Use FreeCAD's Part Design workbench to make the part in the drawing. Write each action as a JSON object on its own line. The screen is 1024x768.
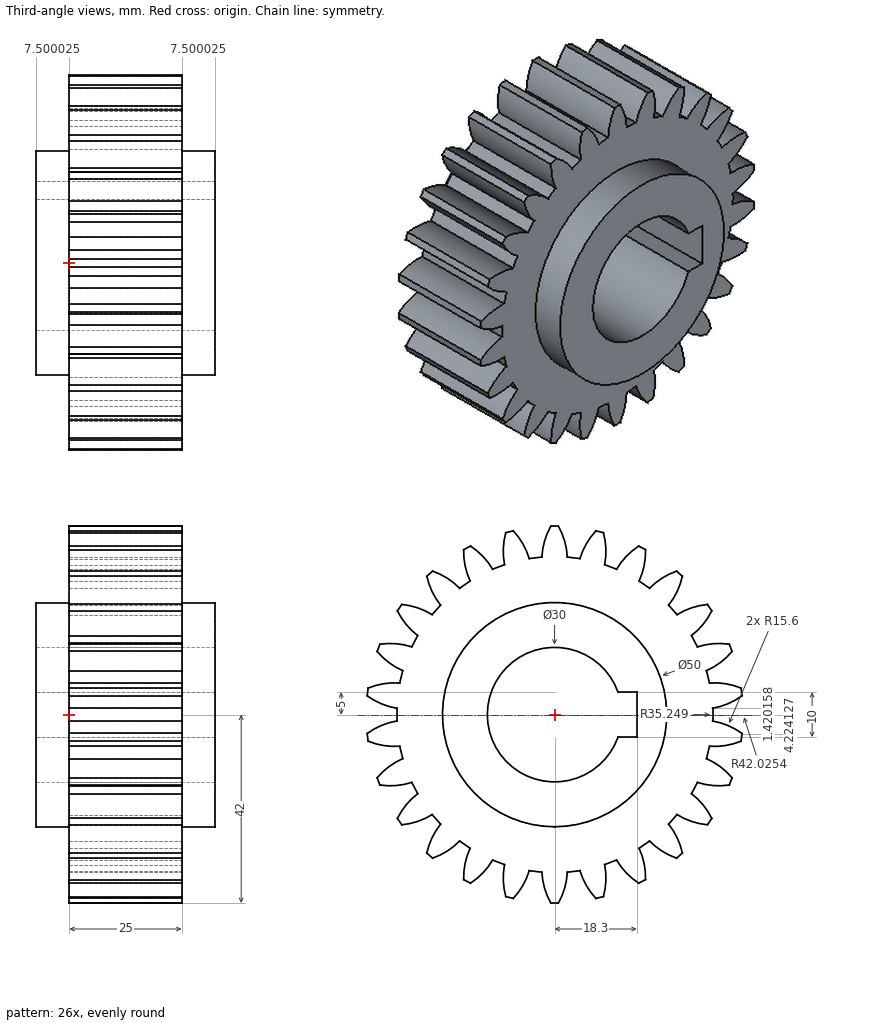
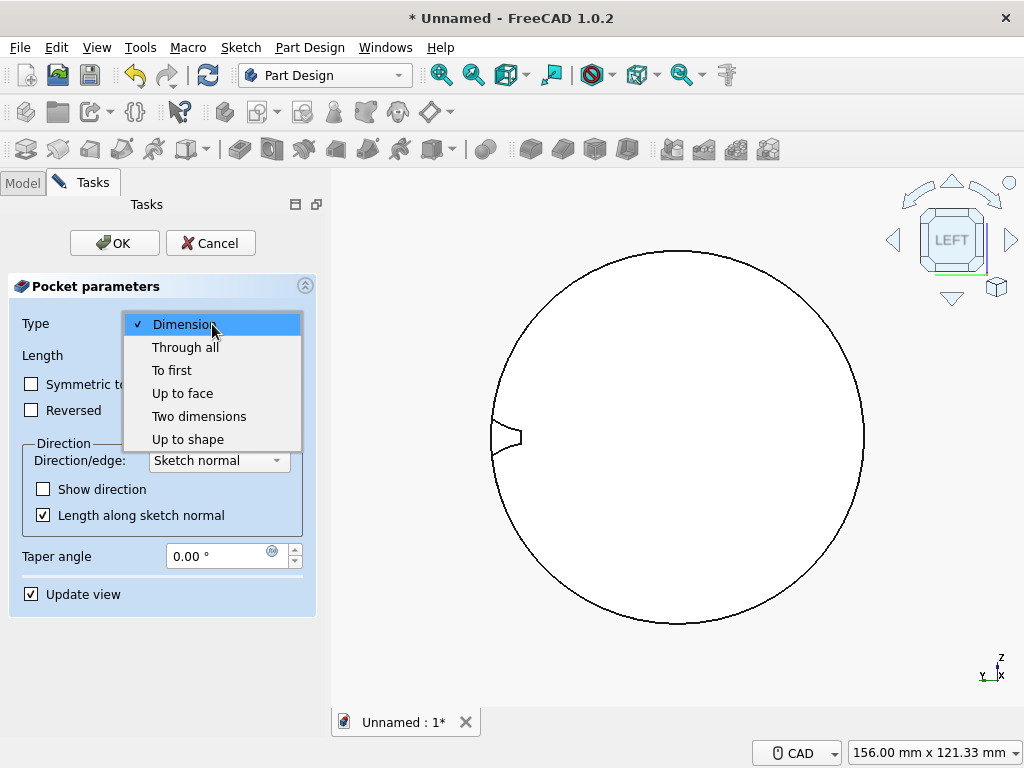
{"action": "left_click", "coordinate": [212, 348]}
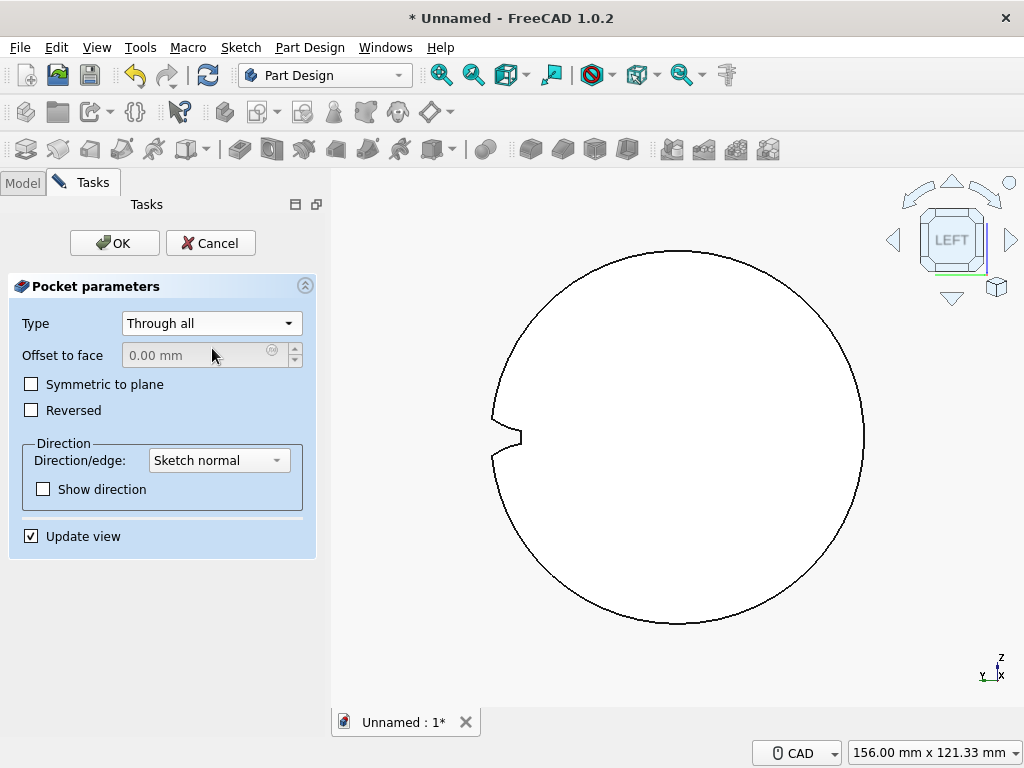
{"action": "left_click", "coordinate": [115, 243]}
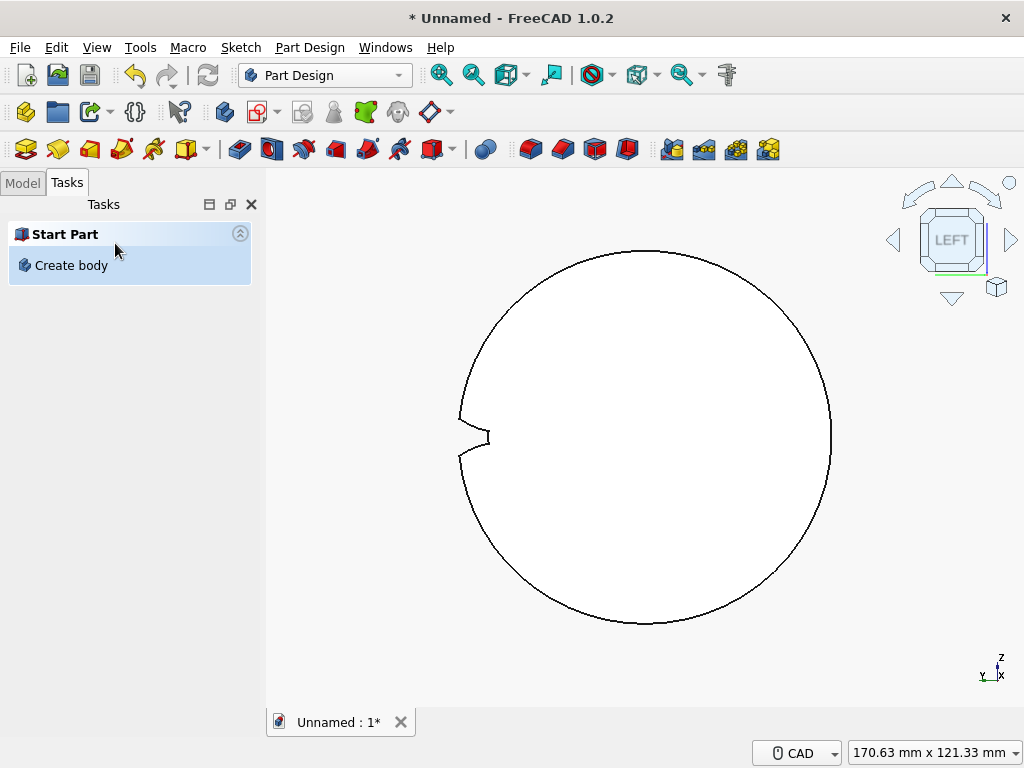
{"action": "left_click", "coordinate": [23, 182]}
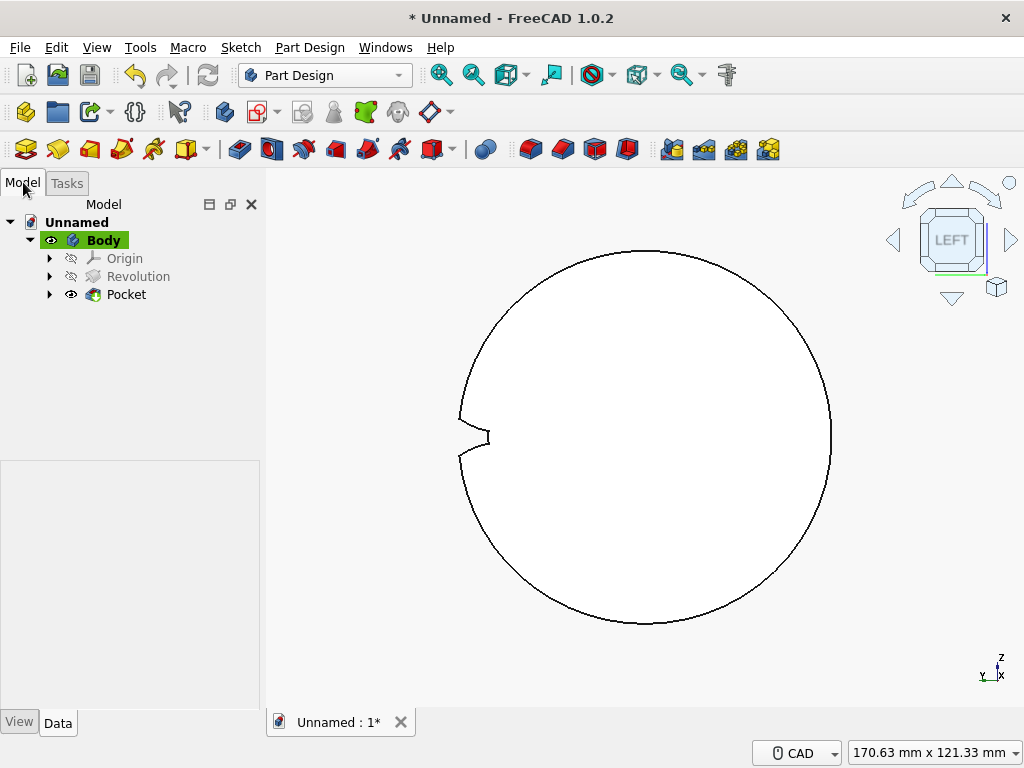
{"action": "left_click", "coordinate": [116, 294]}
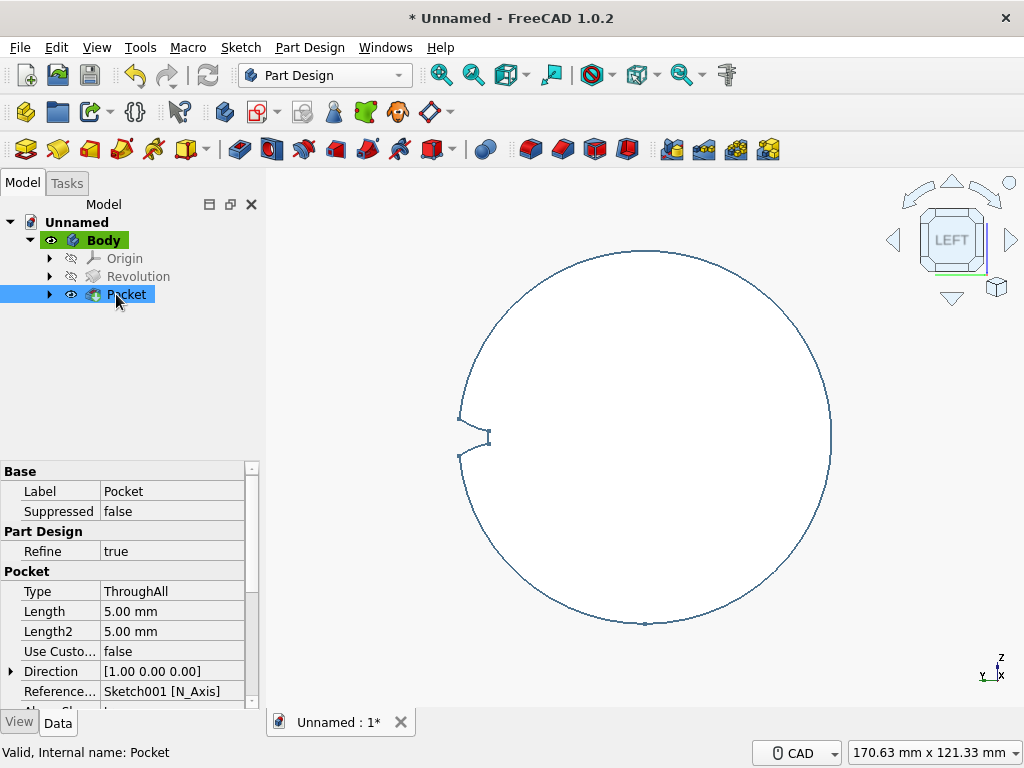
{"action": "left_click", "coordinate": [736, 150]}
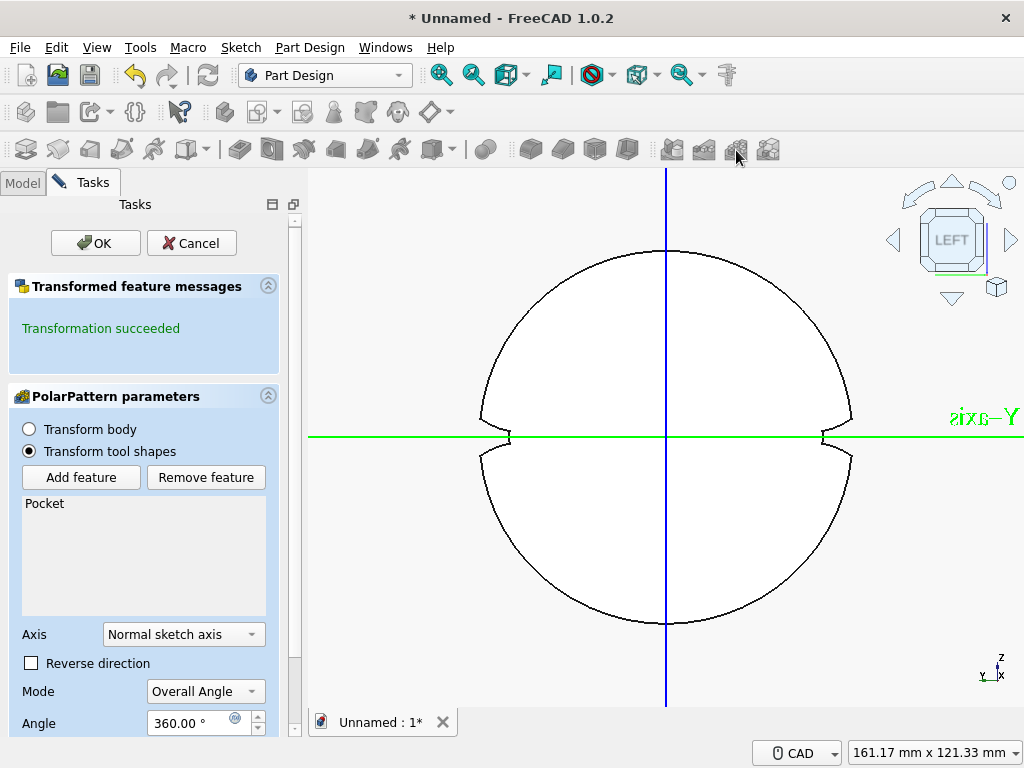
{"action": "left_click", "coordinate": [184, 634]}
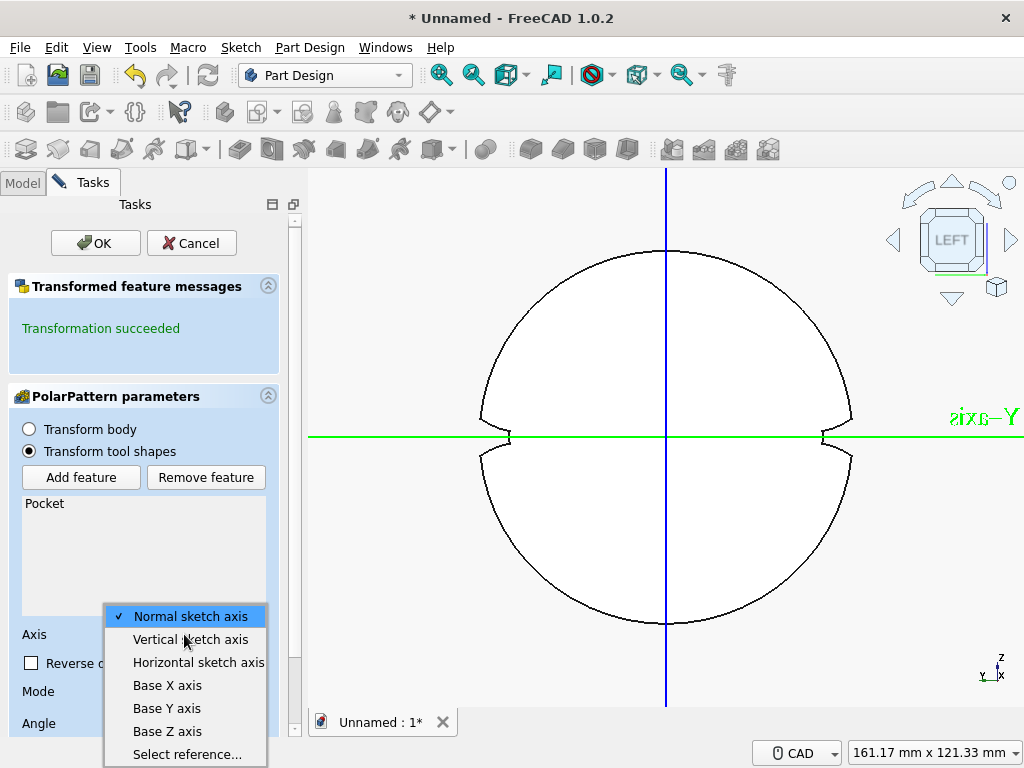
{"action": "left_click", "coordinate": [184, 686]}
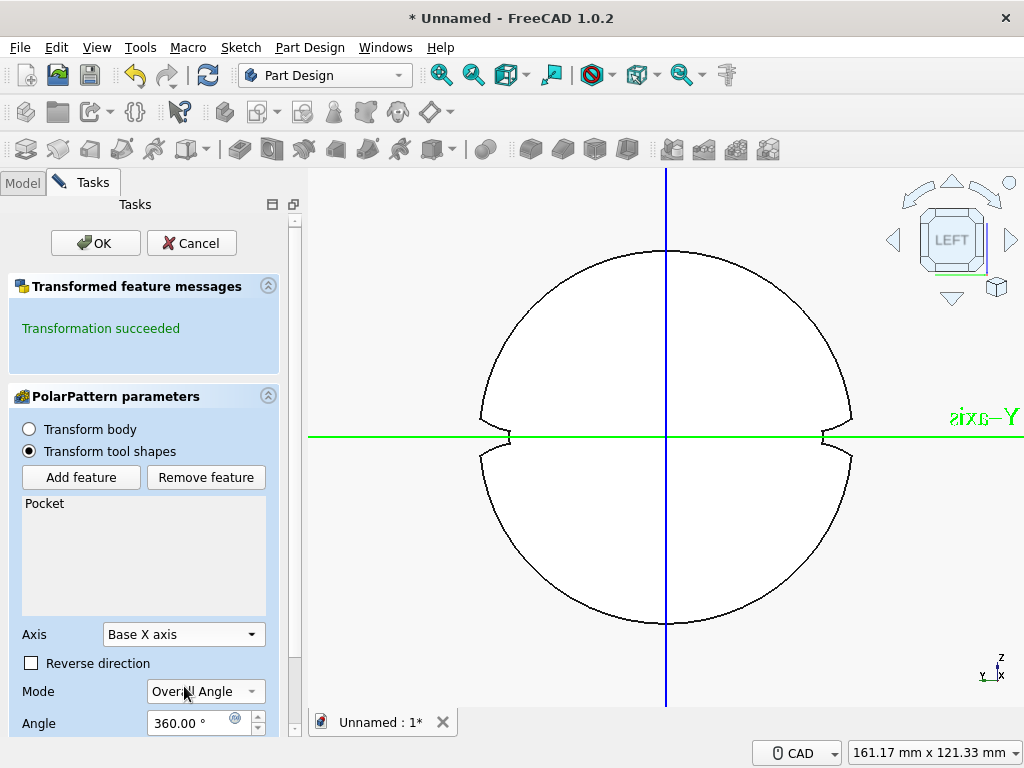
{"action": "scroll", "coordinate": [295, 475], "scroll_direction": "down", "scroll_amount": 2}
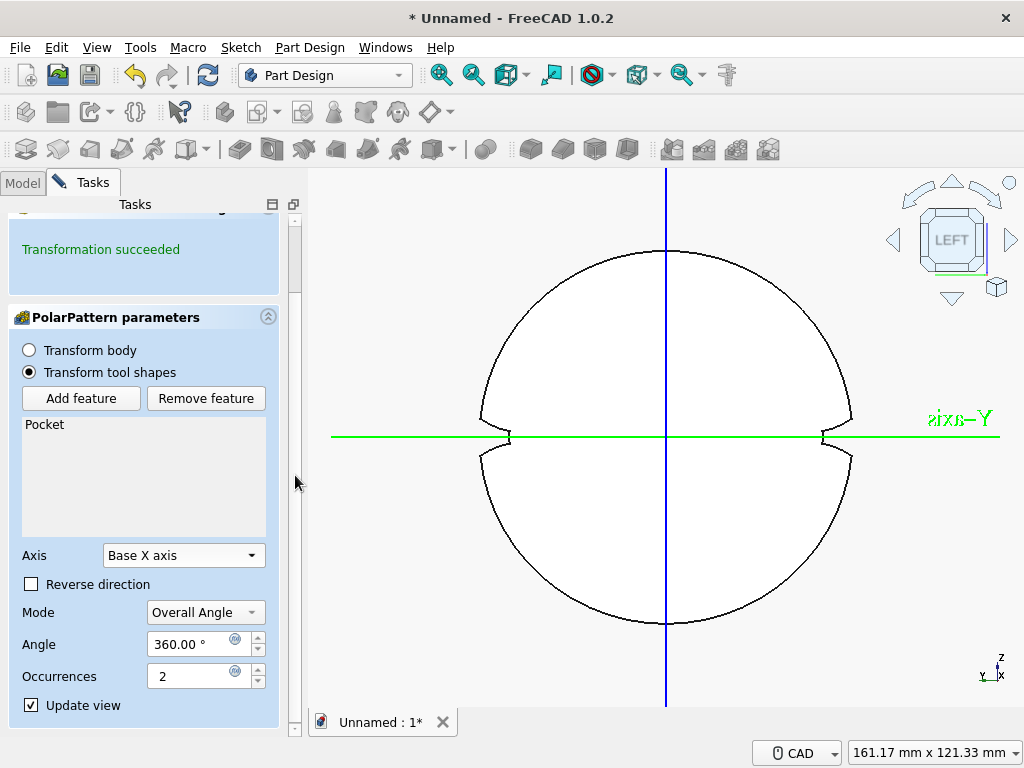
{"action": "triple_click", "coordinate": [198, 676]}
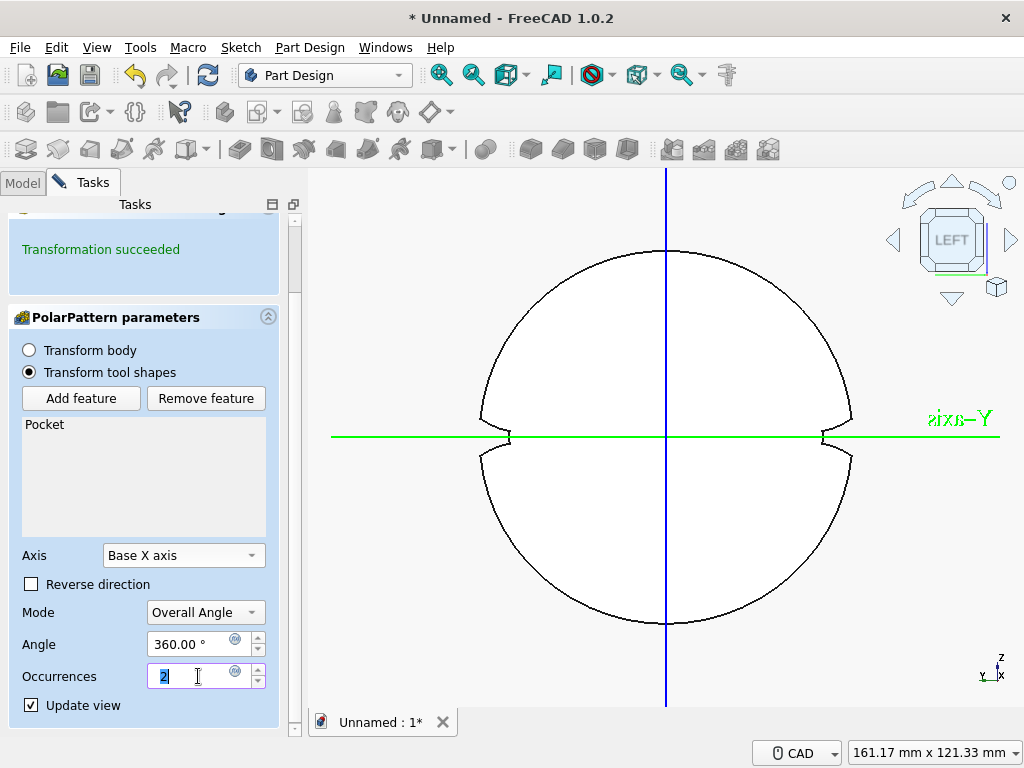
{"action": "type", "text": "26"}
{"action": "key", "text": "Tab"}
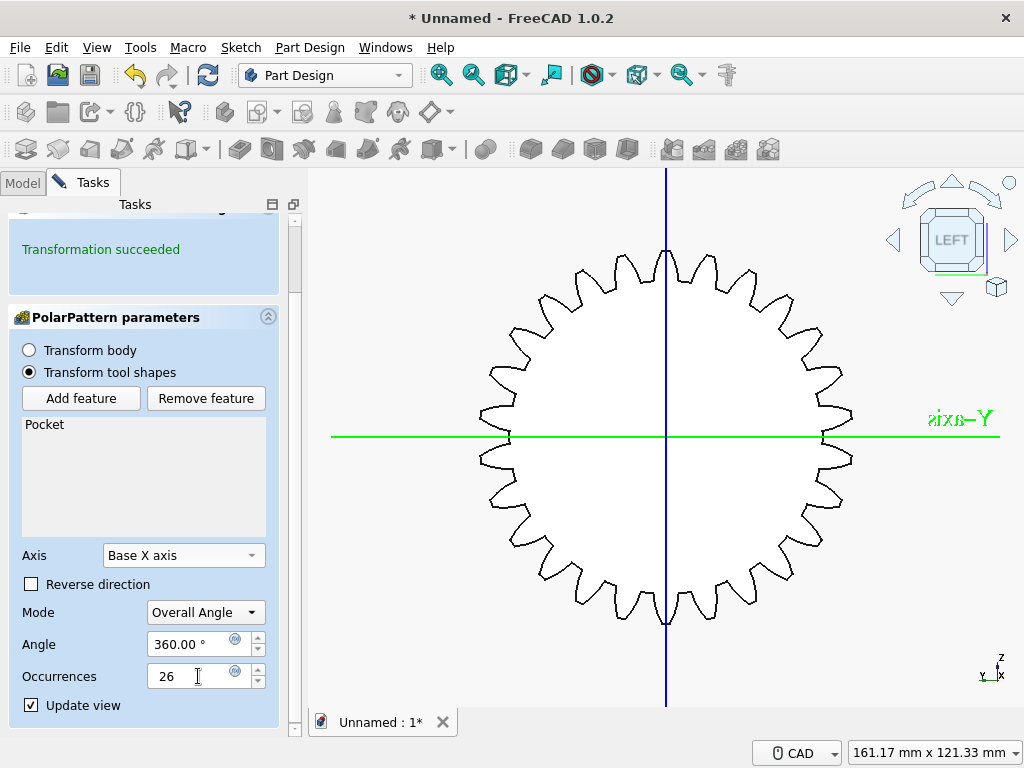
{"action": "scroll", "coordinate": [295, 475], "scroll_direction": "up", "scroll_amount": 3}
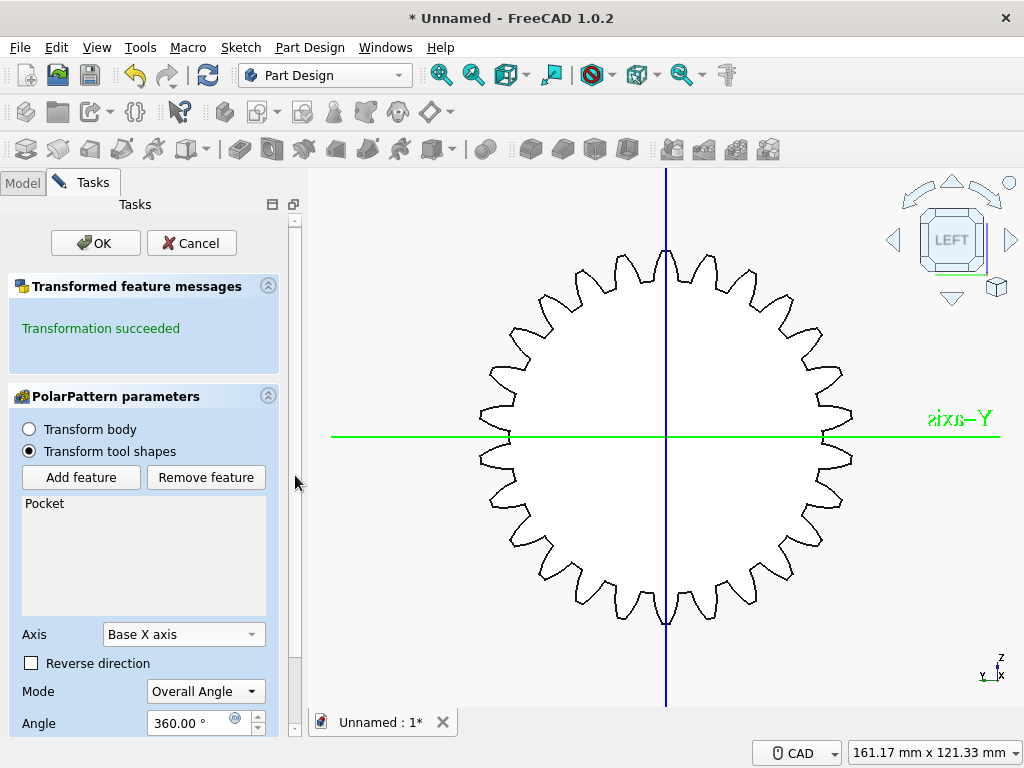
{"action": "left_click", "coordinate": [96, 243]}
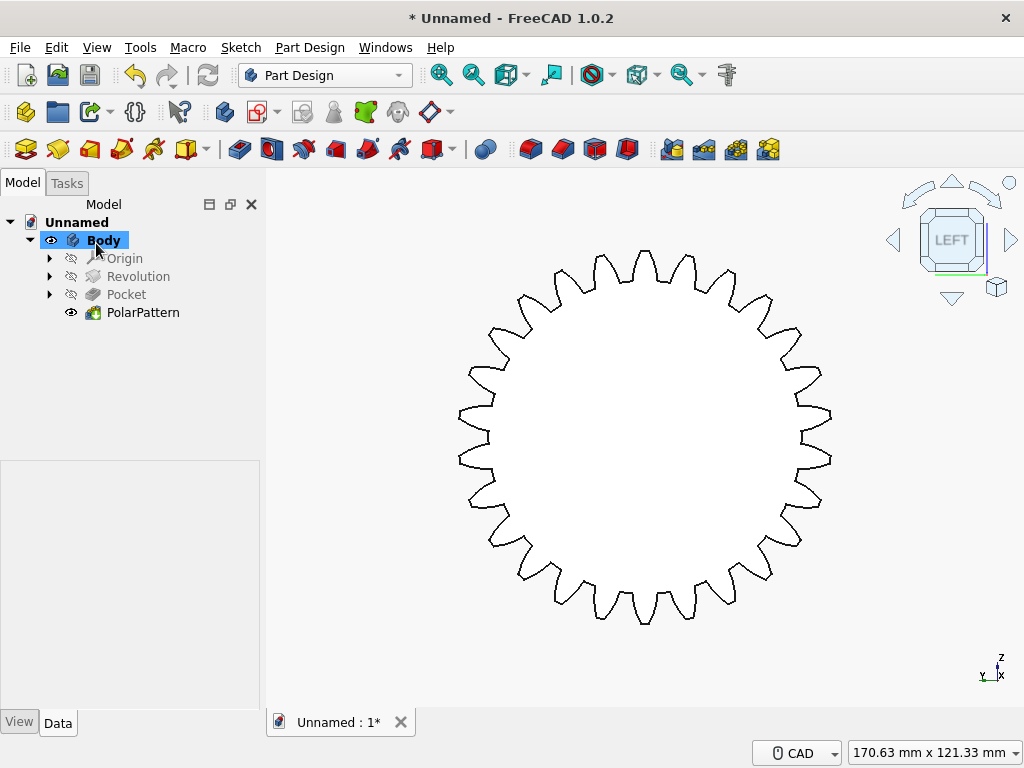
{"action": "left_click", "coordinate": [258, 112]}